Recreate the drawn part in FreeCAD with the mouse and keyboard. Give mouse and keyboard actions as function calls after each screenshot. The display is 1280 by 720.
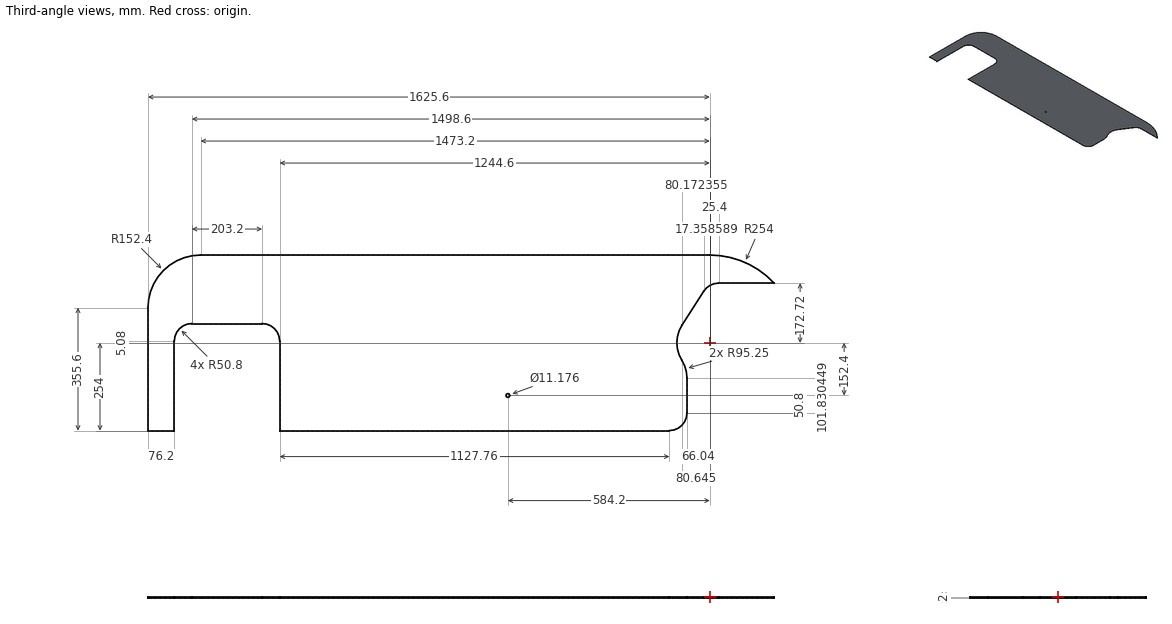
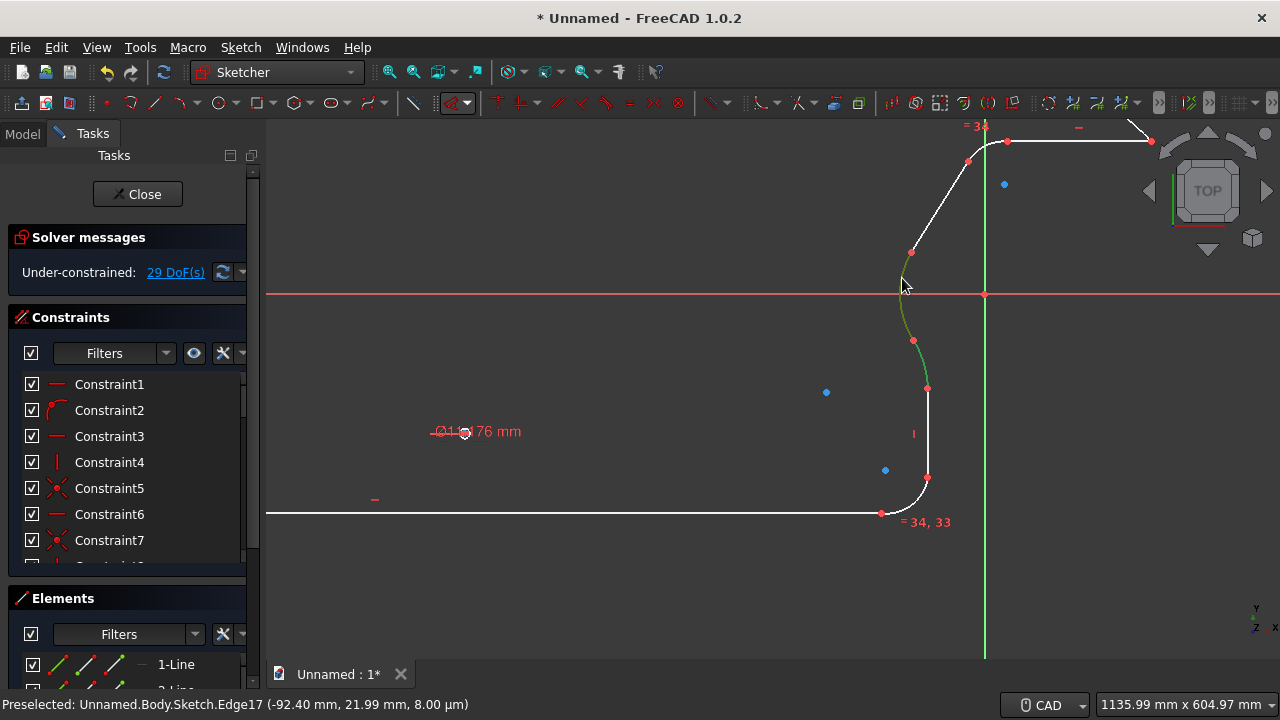
click(630, 104)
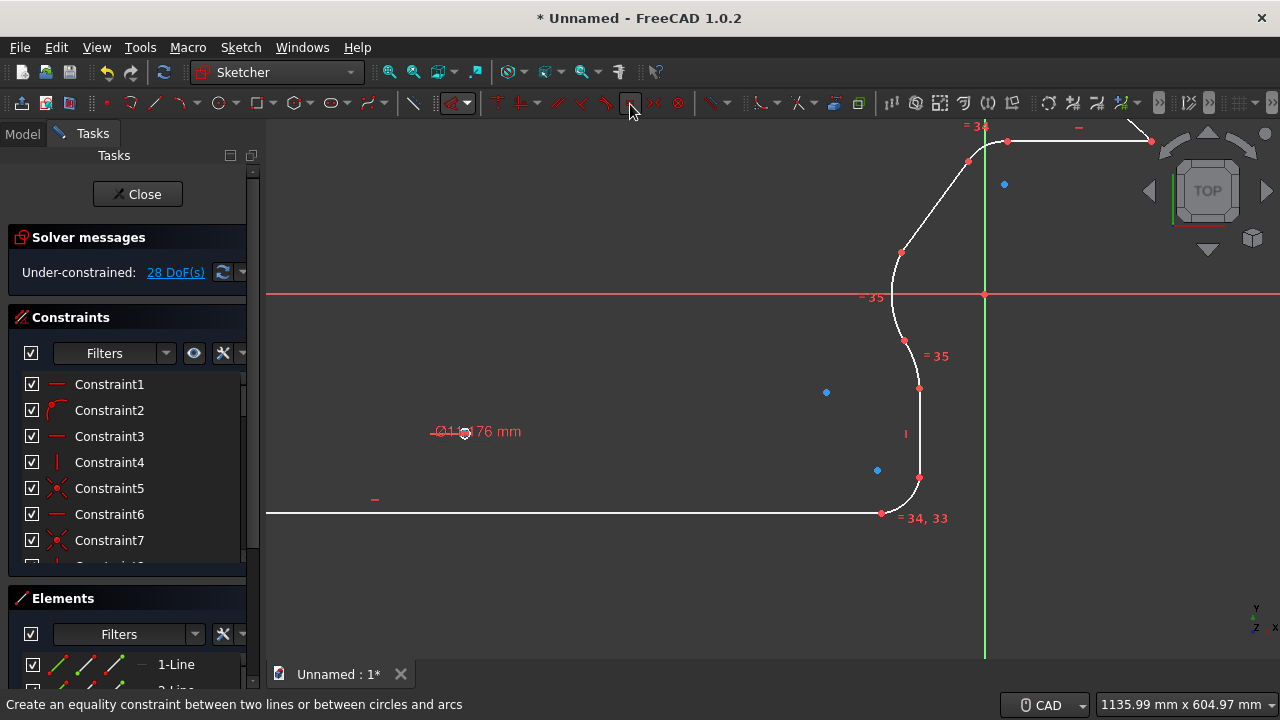
click(452, 104)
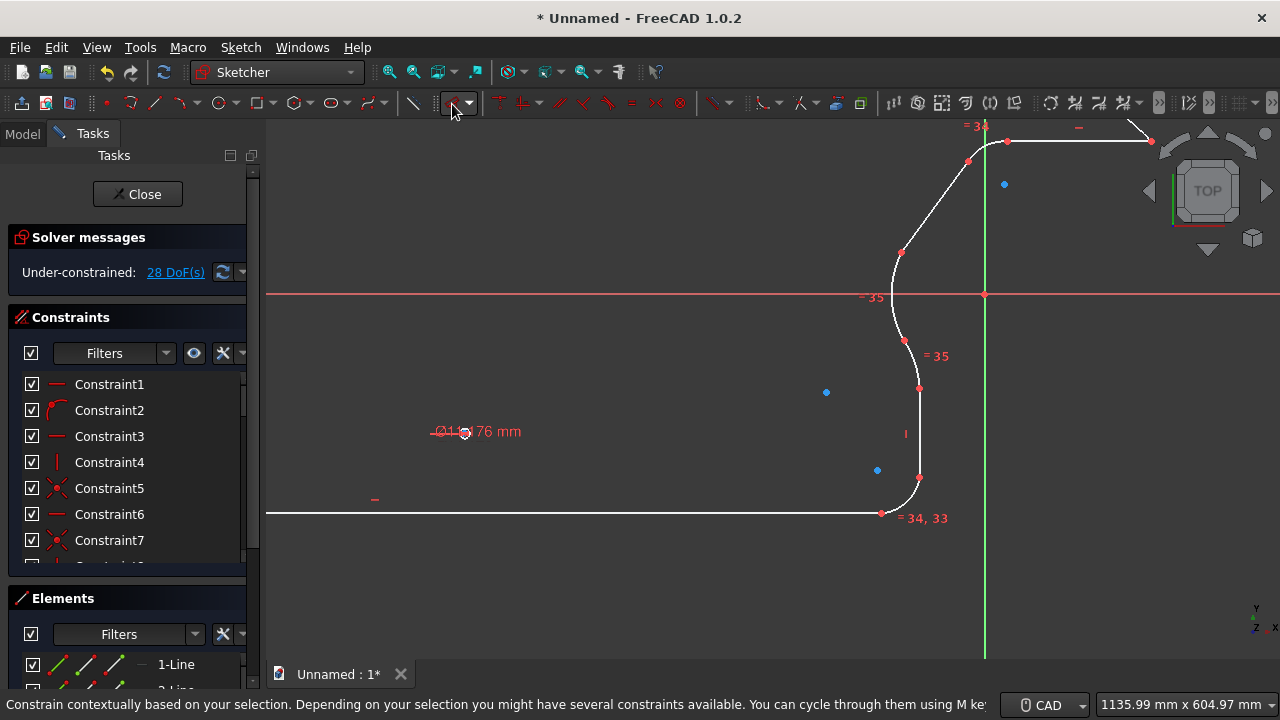
scroll(915, 444, down, 5)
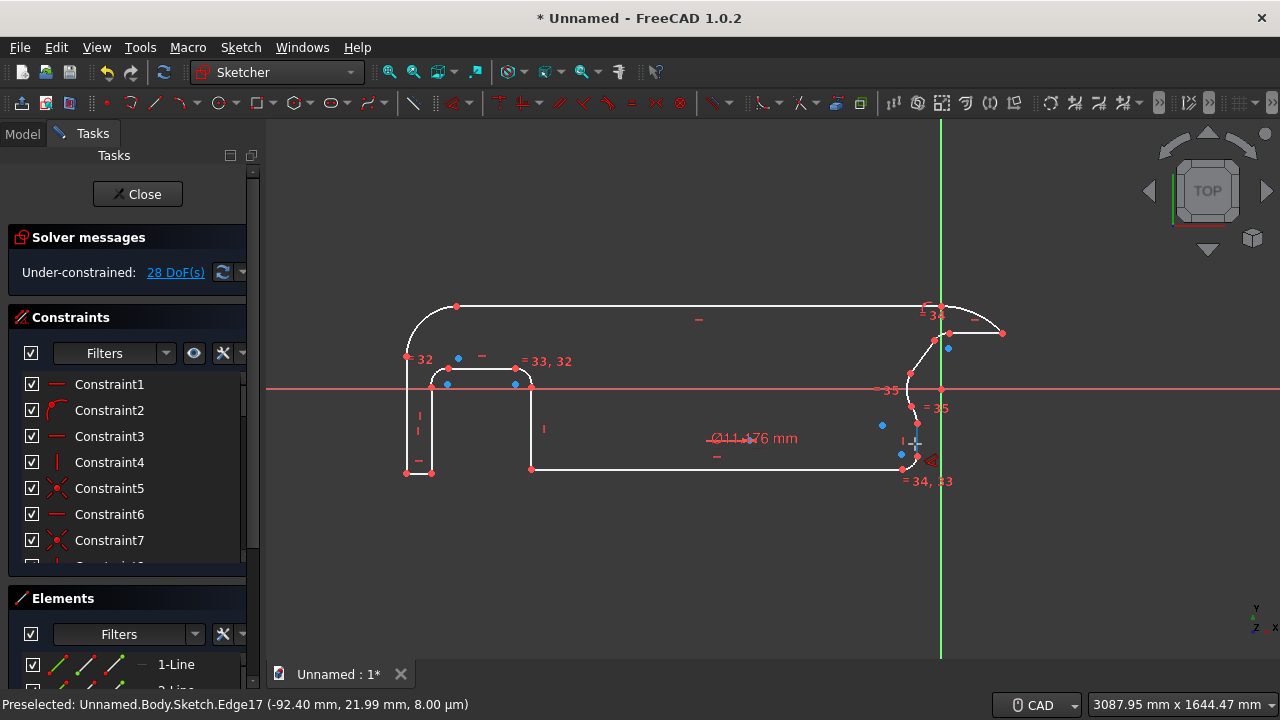
click(987, 320)
click(1005, 293)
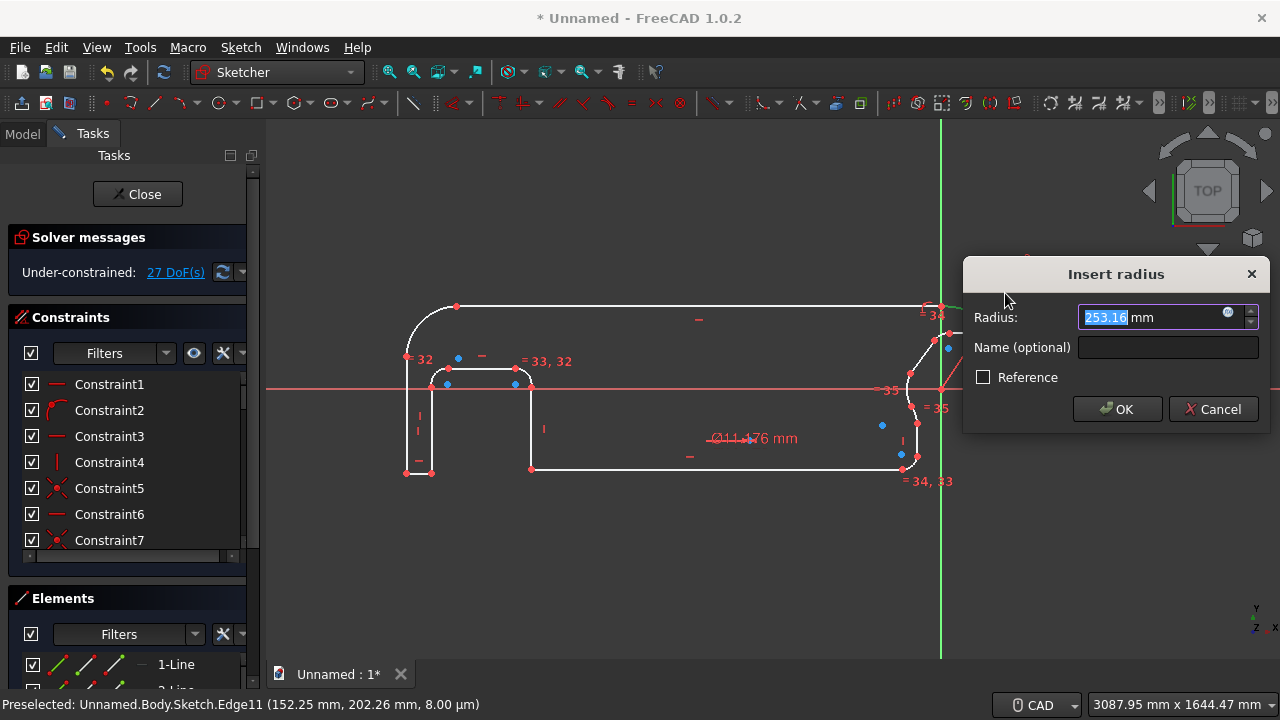
text(254)
key(Return)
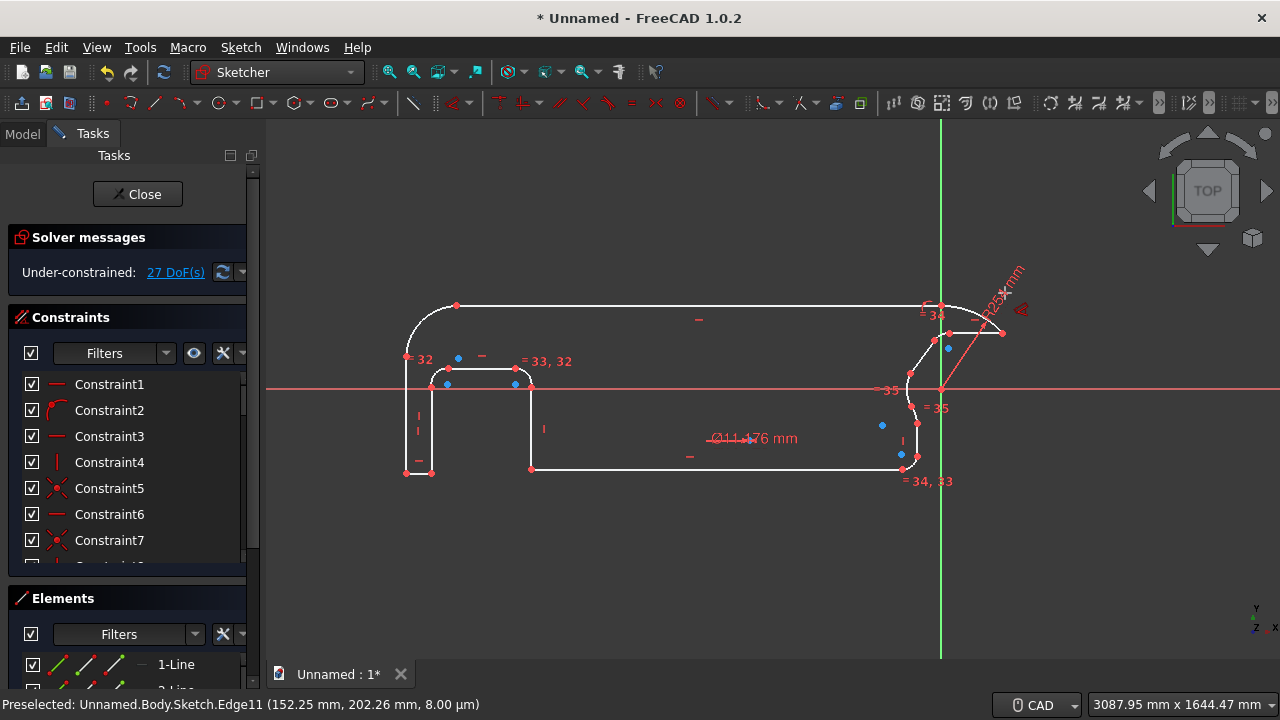
click(434, 312)
click(419, 284)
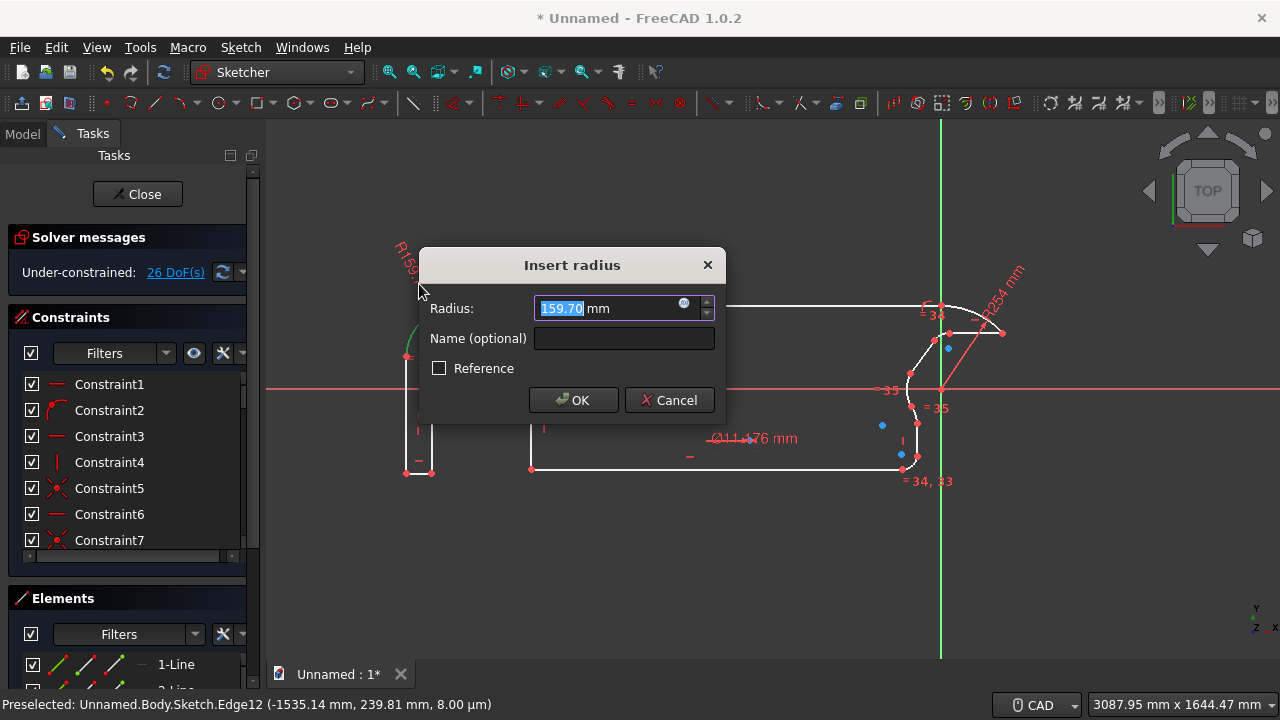
text(152.4)
key(Return)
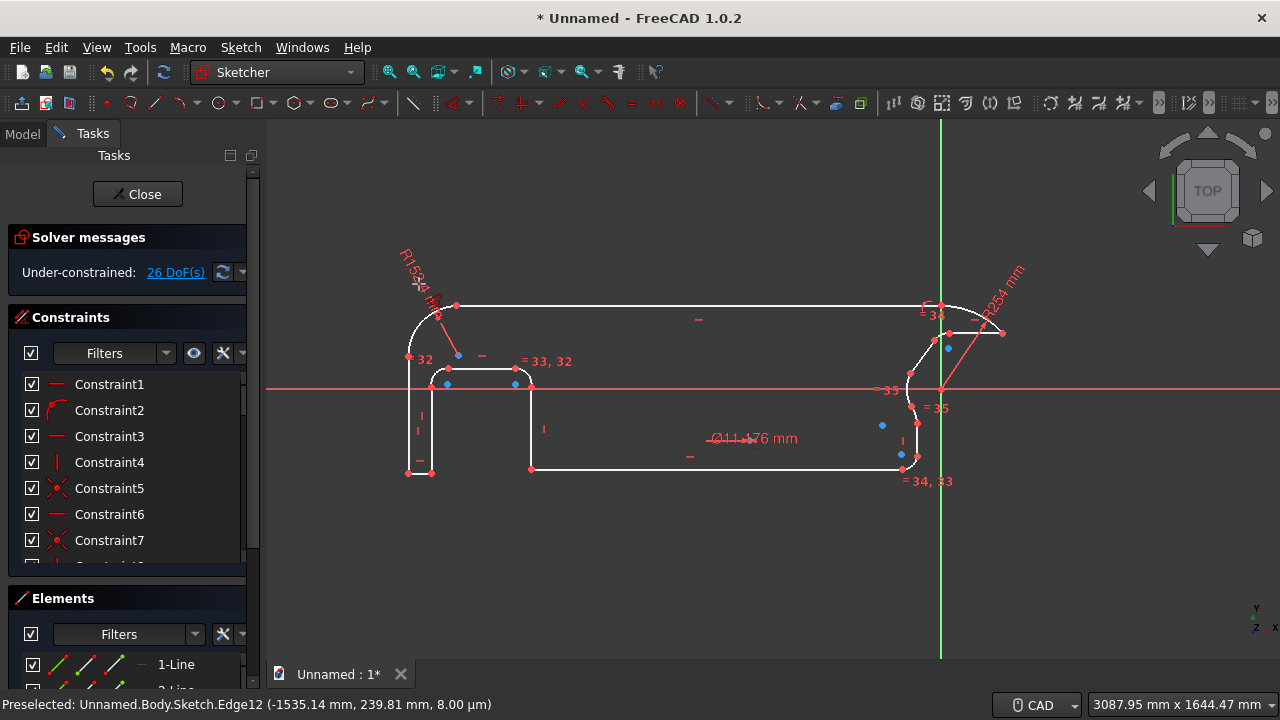
scroll(435, 374, up, 5)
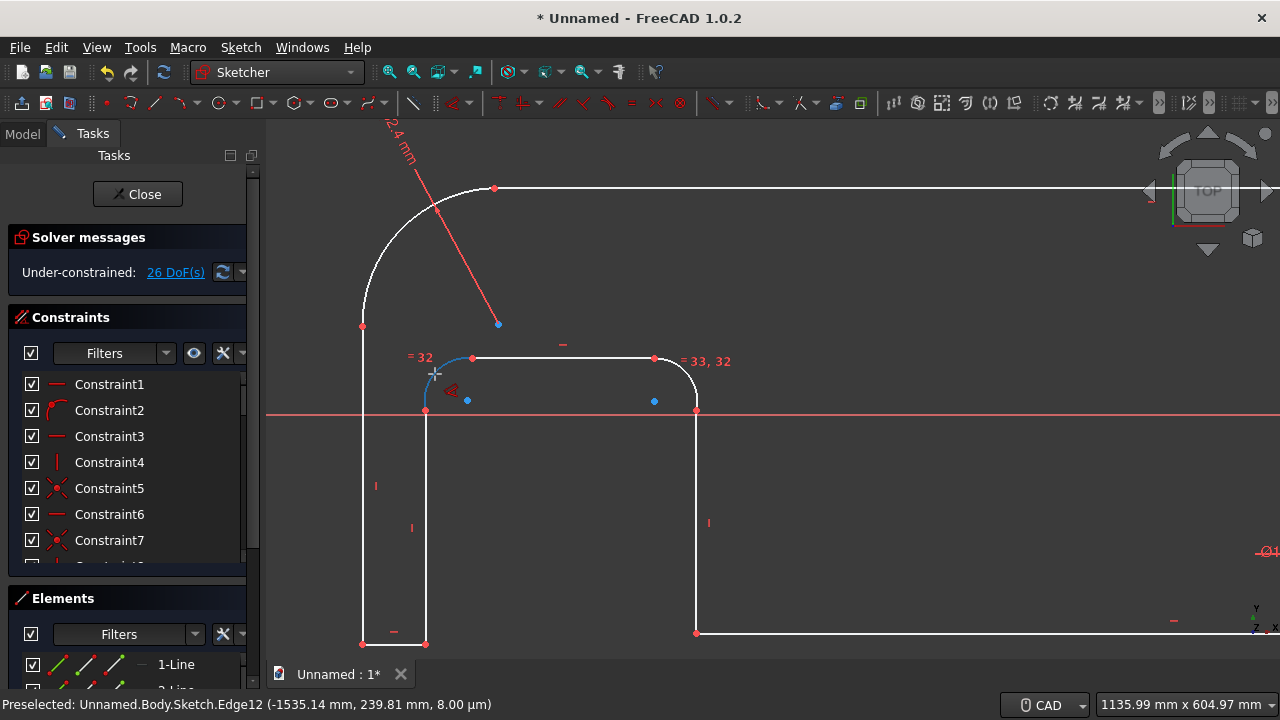
click(436, 372)
click(412, 350)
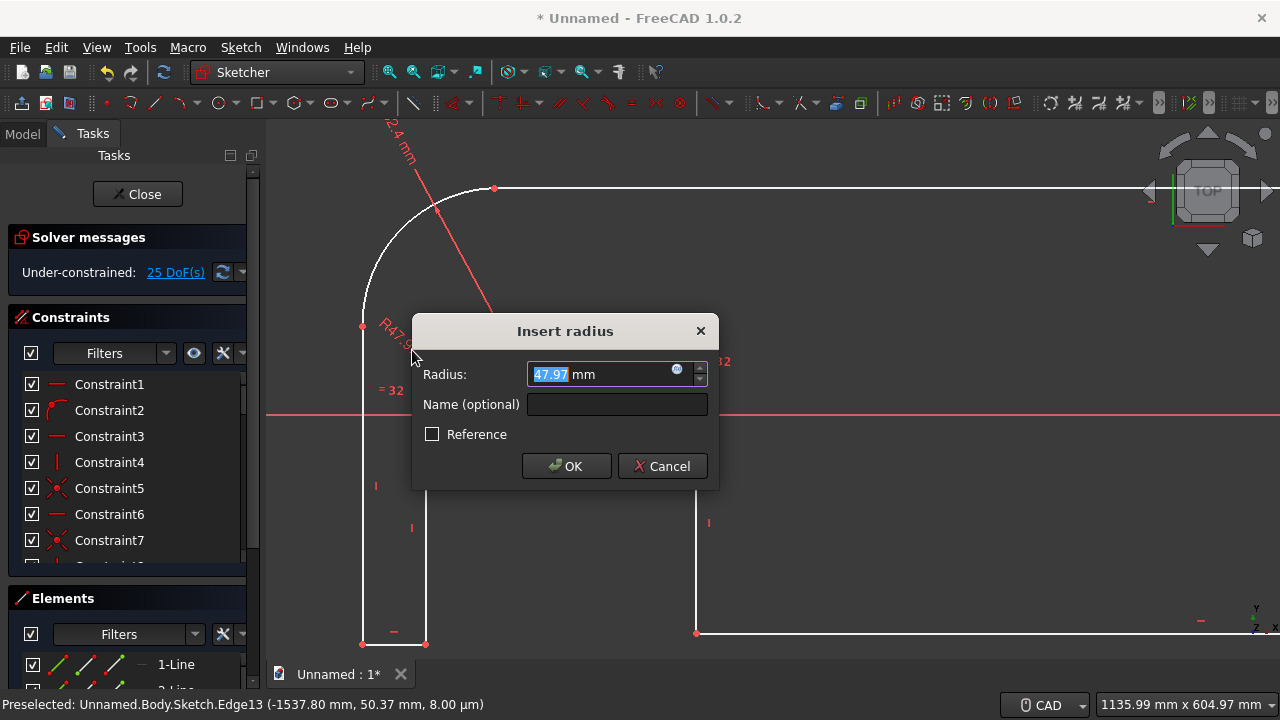
text(50.8)
key(Return)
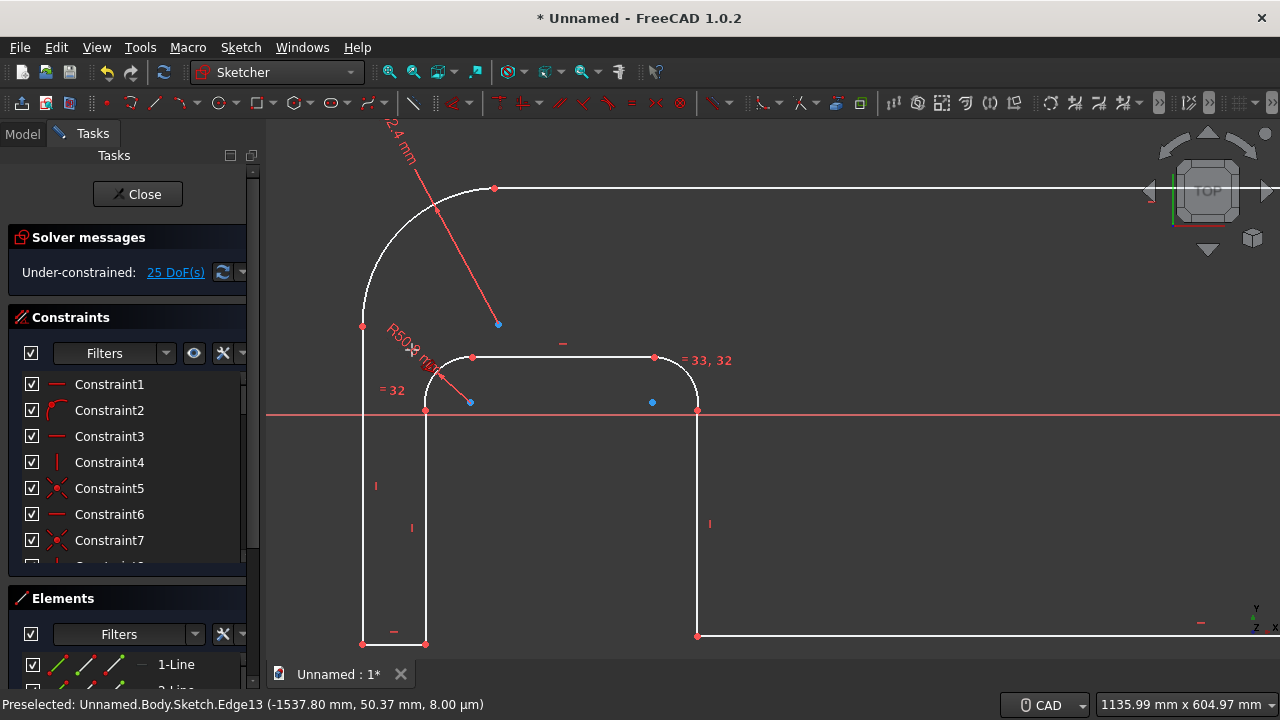
scroll(435, 374, down, 5)